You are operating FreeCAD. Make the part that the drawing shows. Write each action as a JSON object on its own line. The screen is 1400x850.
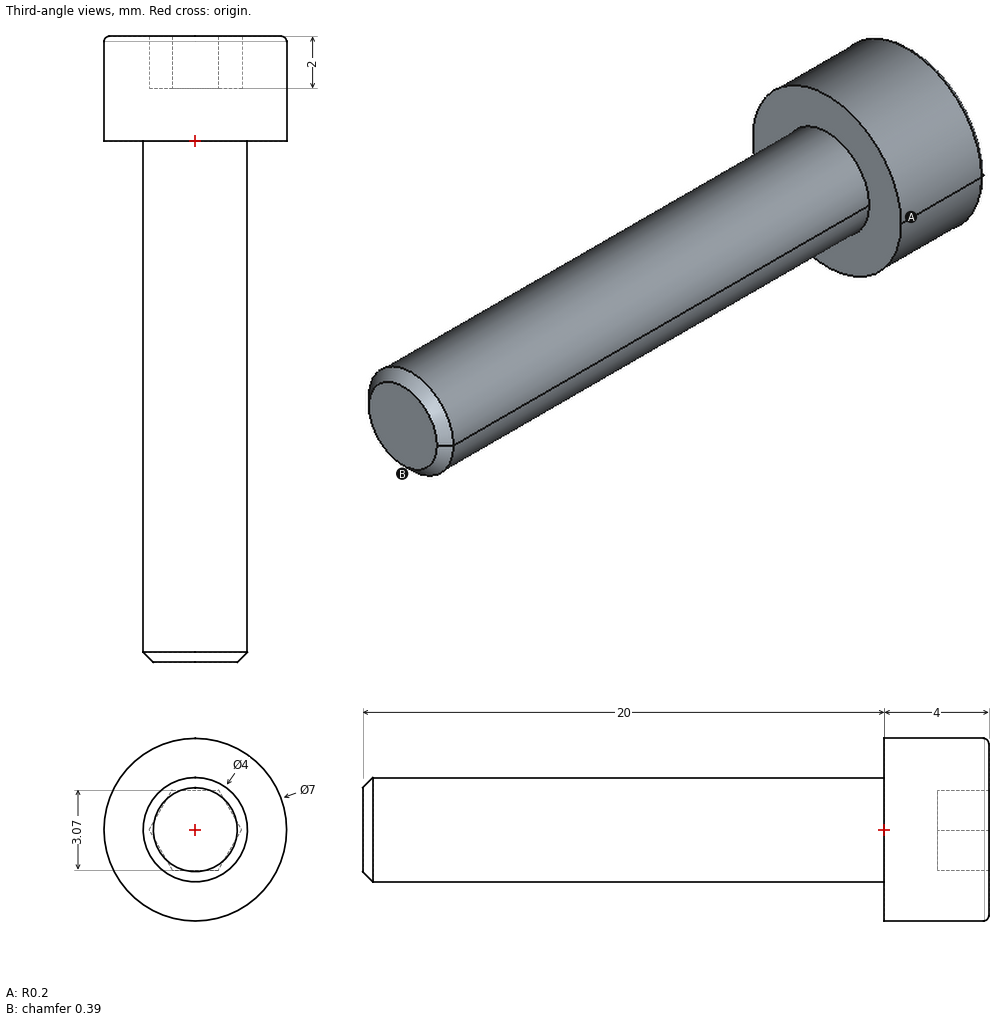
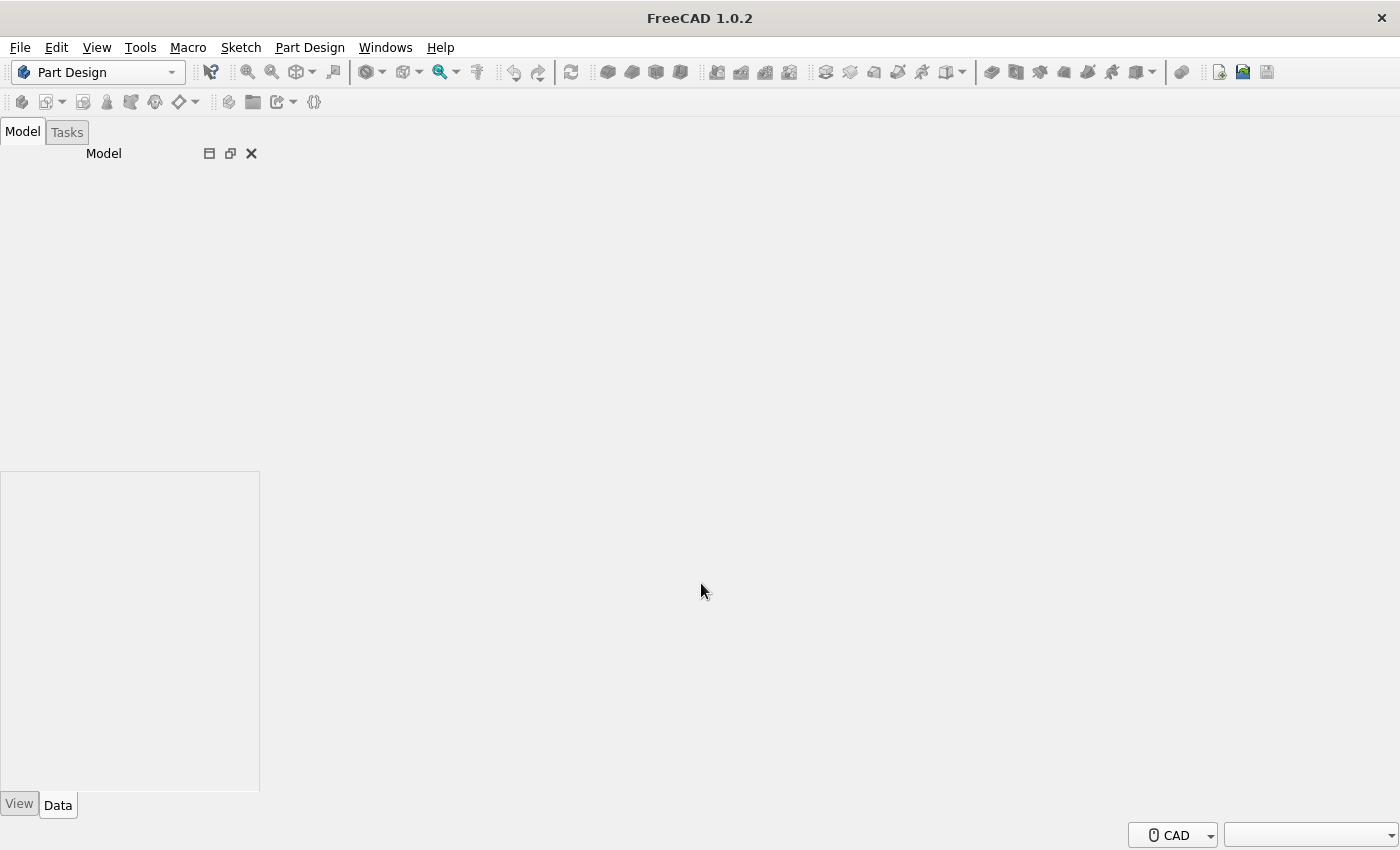
{"action": "key", "text": "ctrl+n"}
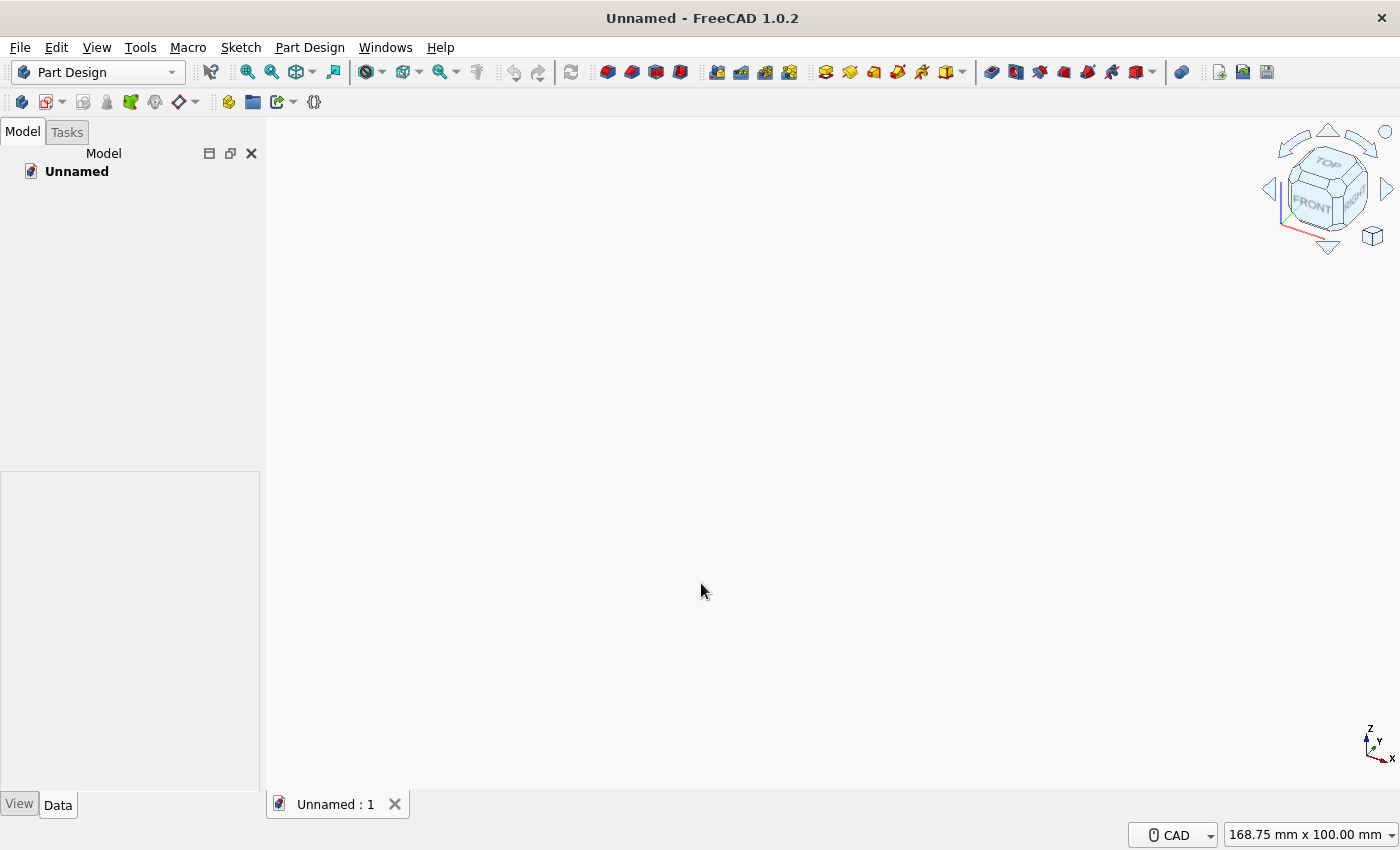
{"action": "left_click", "coordinate": [46, 102]}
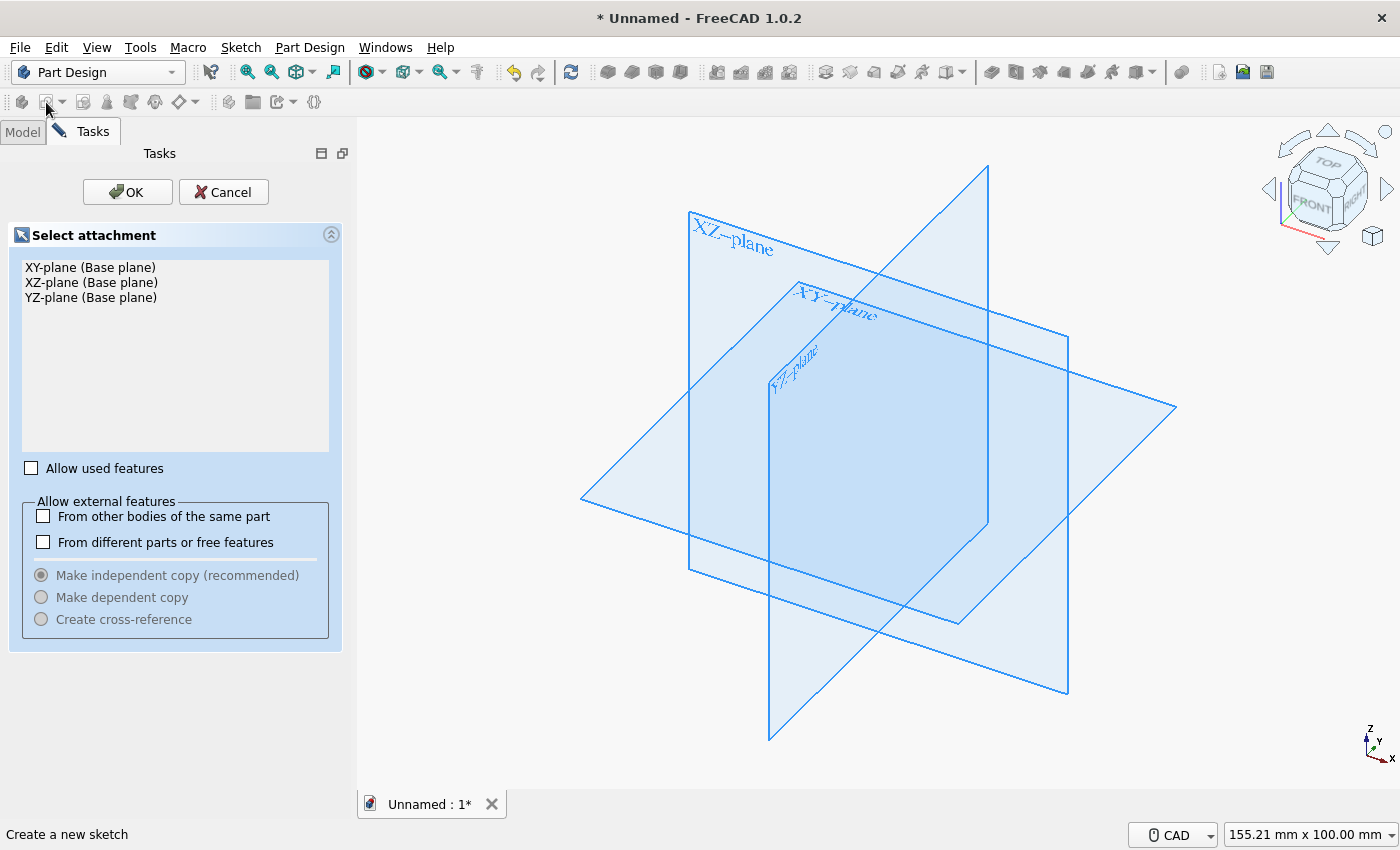
{"action": "left_click", "coordinate": [82, 282]}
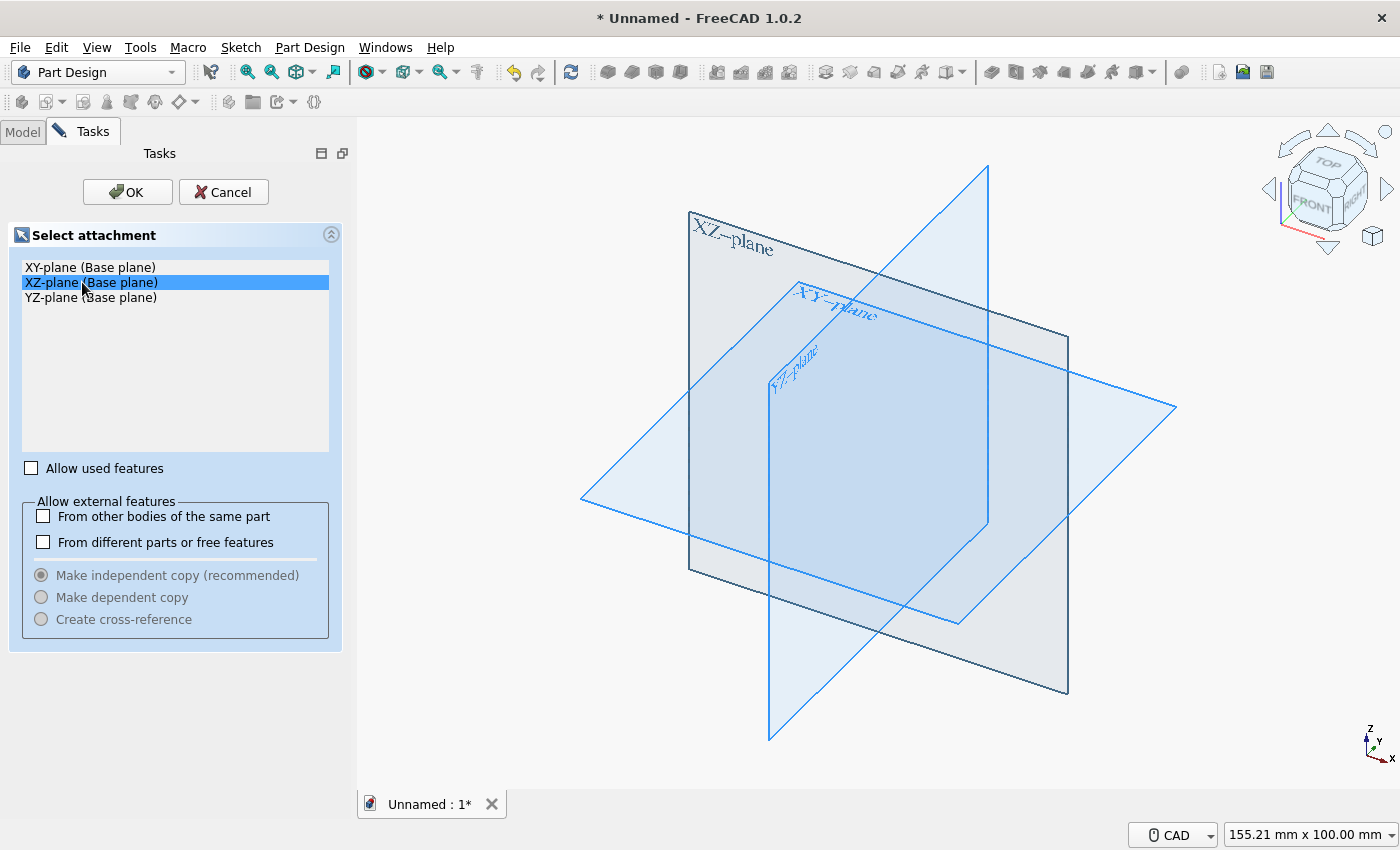
{"action": "left_click", "coordinate": [128, 192]}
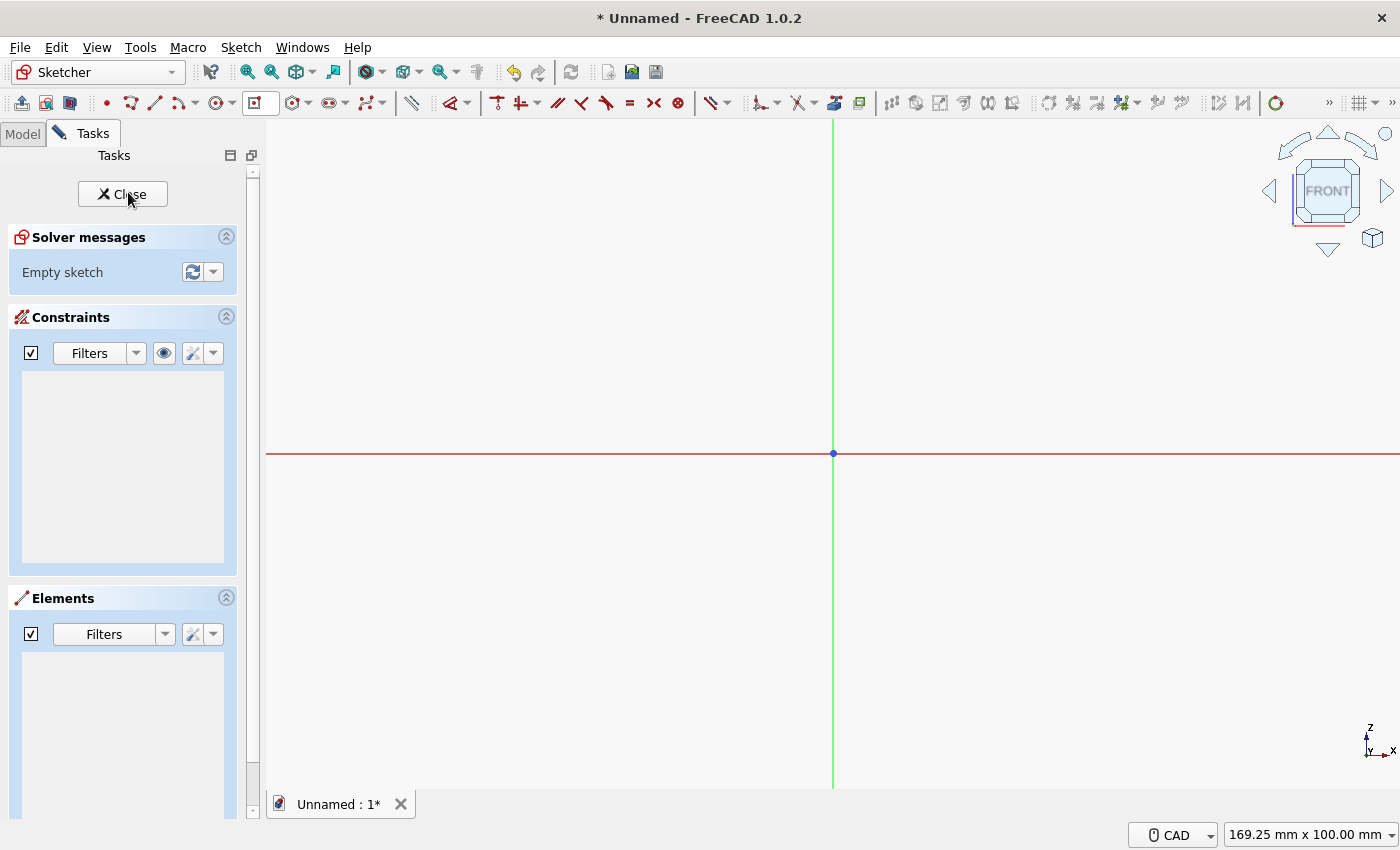
{"action": "scroll", "coordinate": [842, 454], "scroll_direction": "up", "scroll_amount": 11}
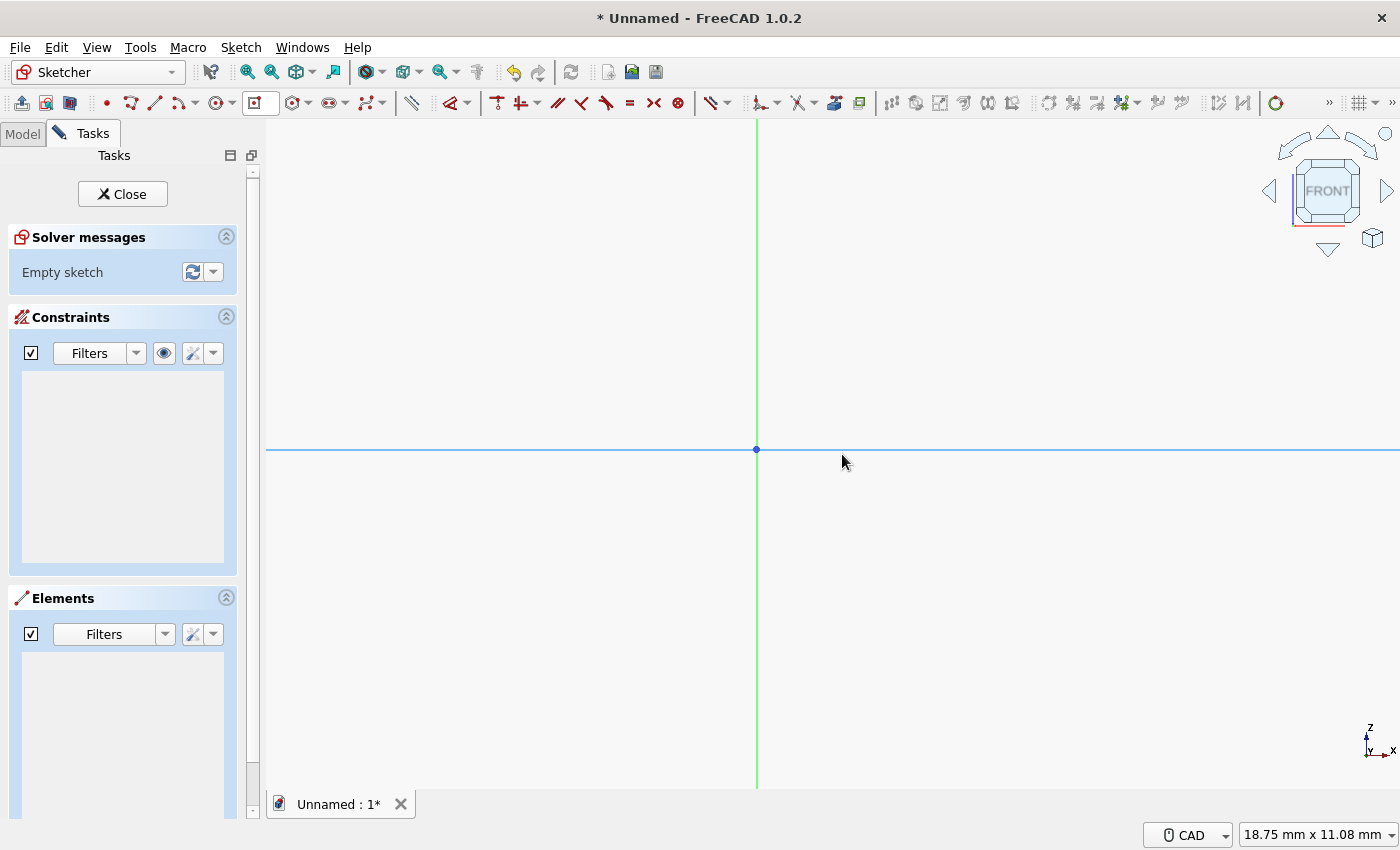
{"action": "key", "text": "g c"}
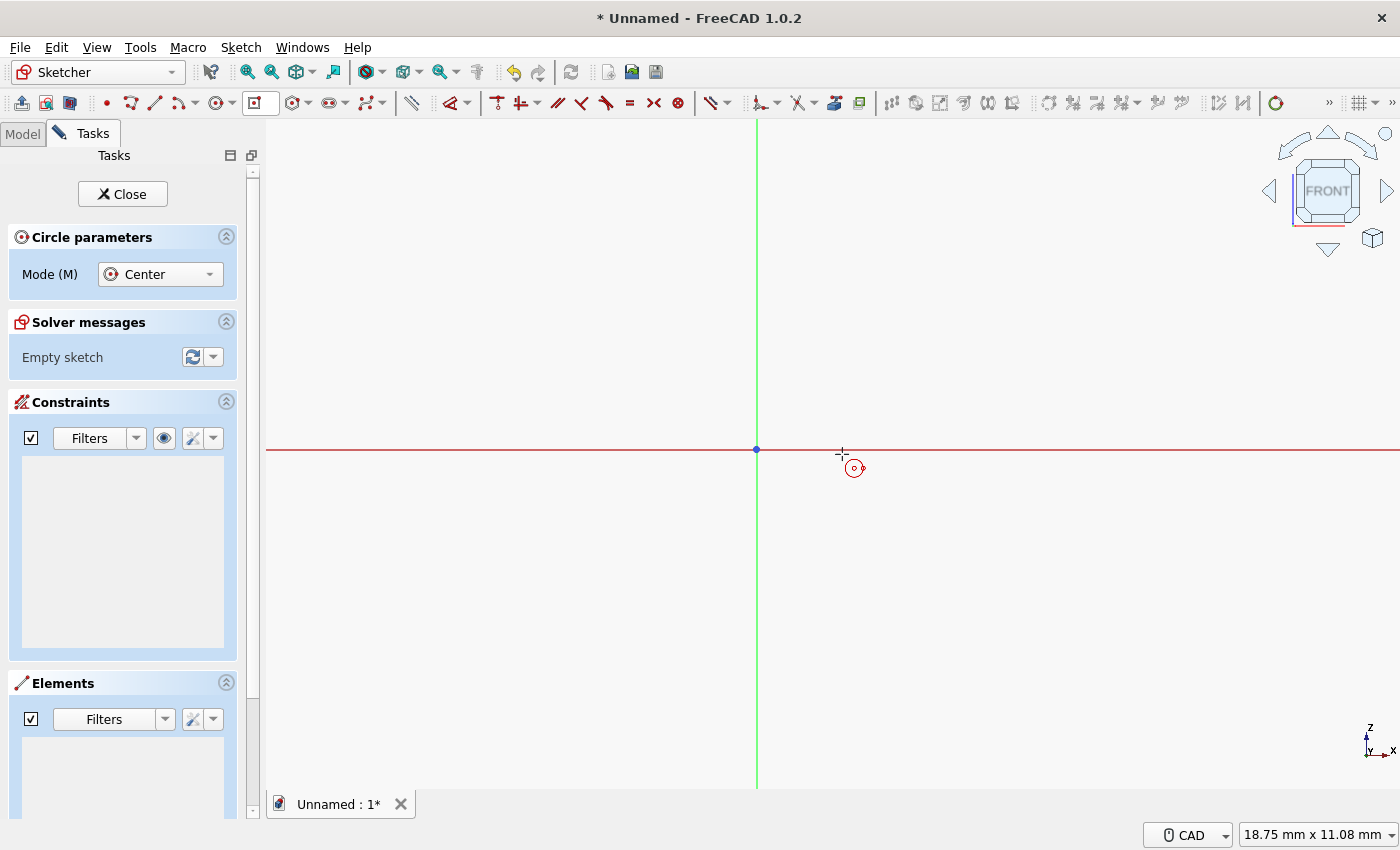
{"action": "left_click", "coordinate": [757, 450]}
{"action": "left_click", "coordinate": [906, 300]}
{"action": "key", "text": "Escape"}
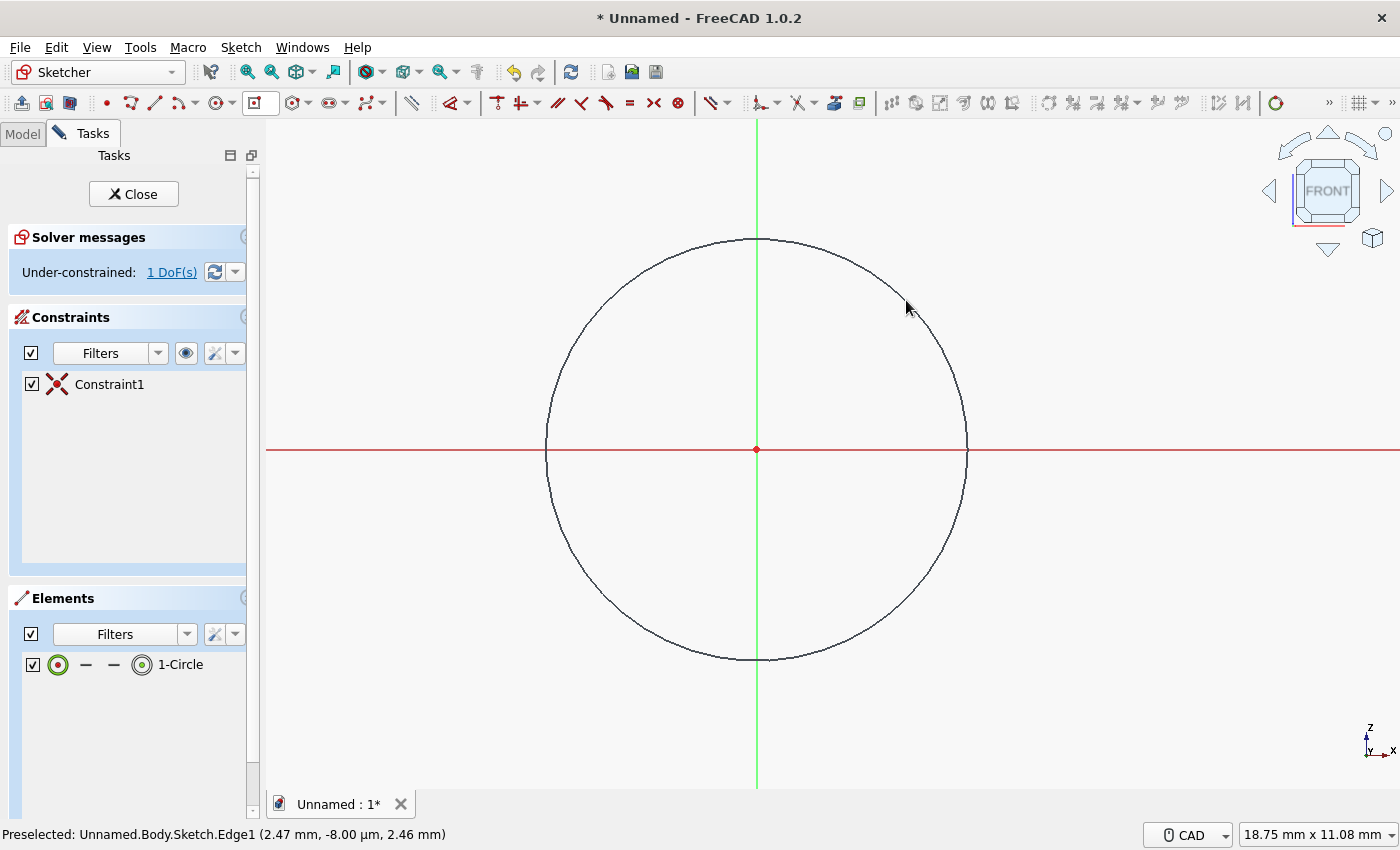
{"action": "key", "text": "d"}